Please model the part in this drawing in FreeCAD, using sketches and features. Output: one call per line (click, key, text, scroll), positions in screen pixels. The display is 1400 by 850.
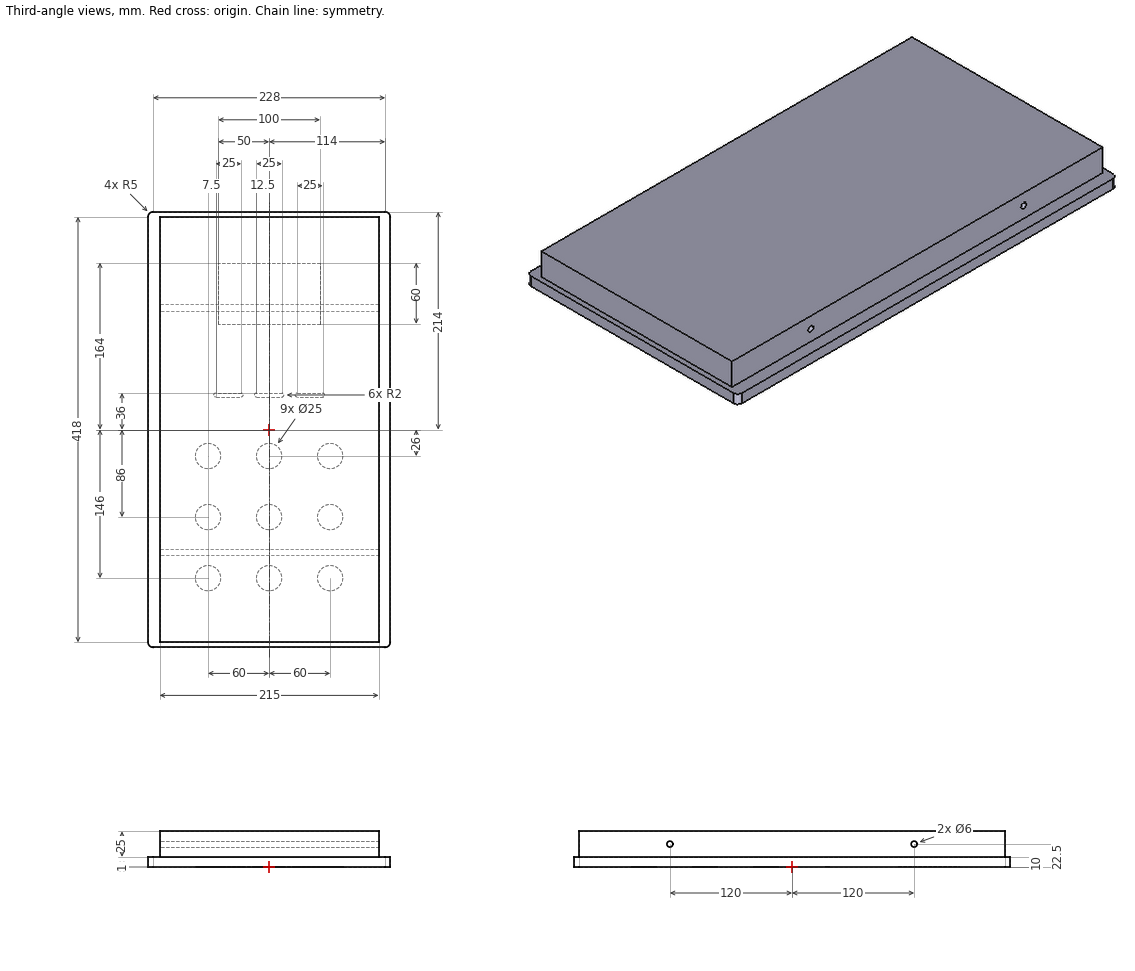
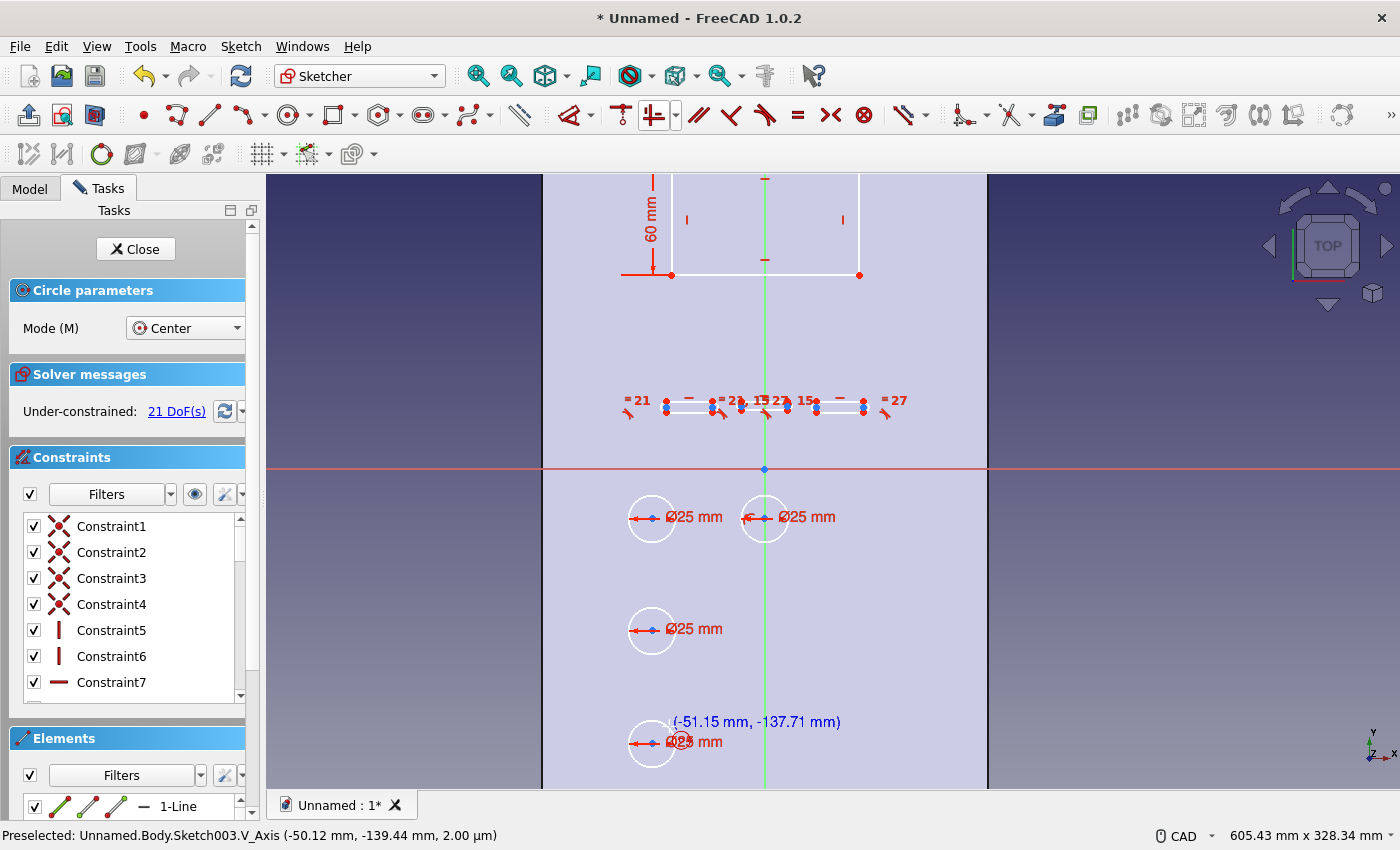
click(765, 630)
move(781, 614)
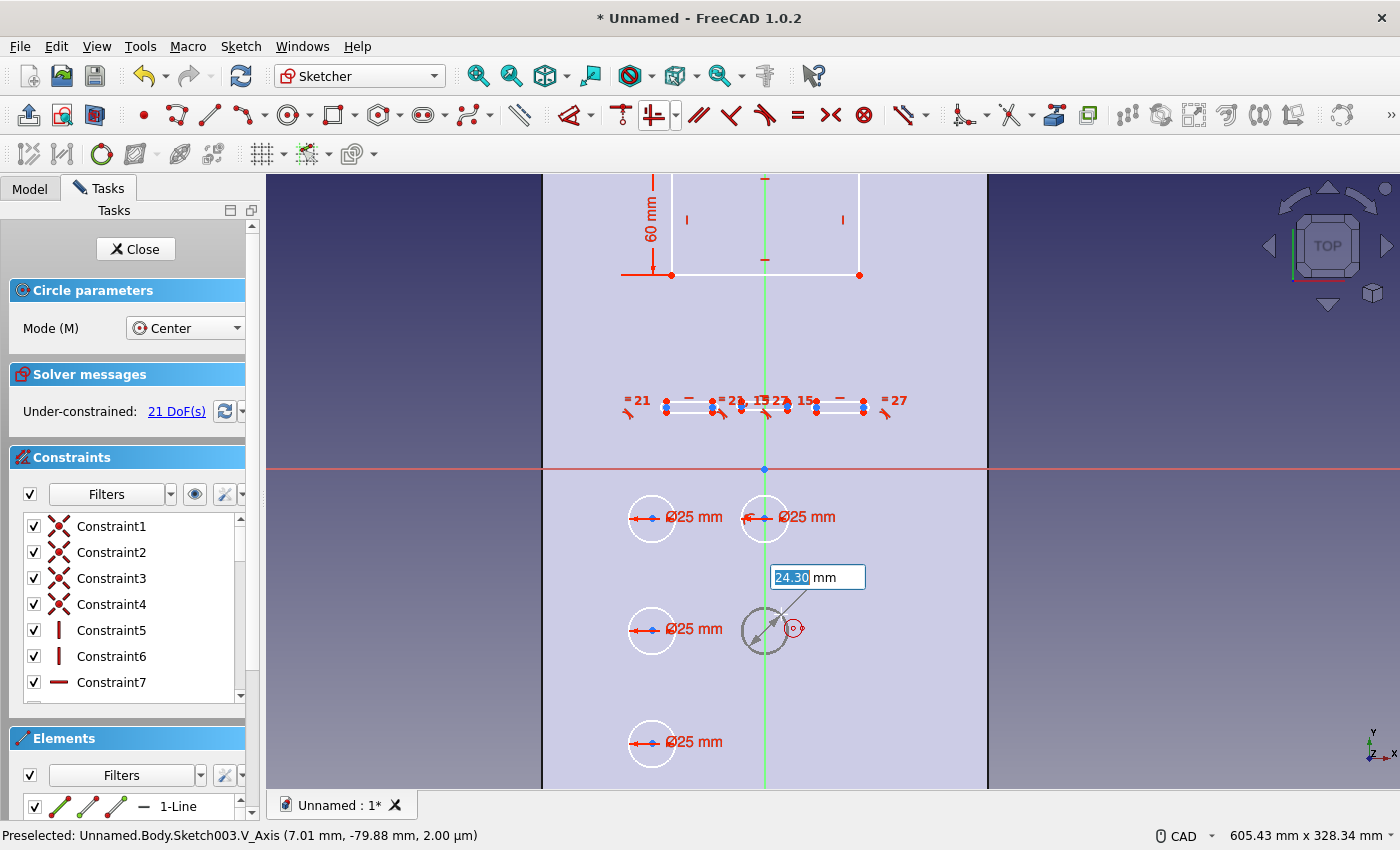
text(25)
key(Return)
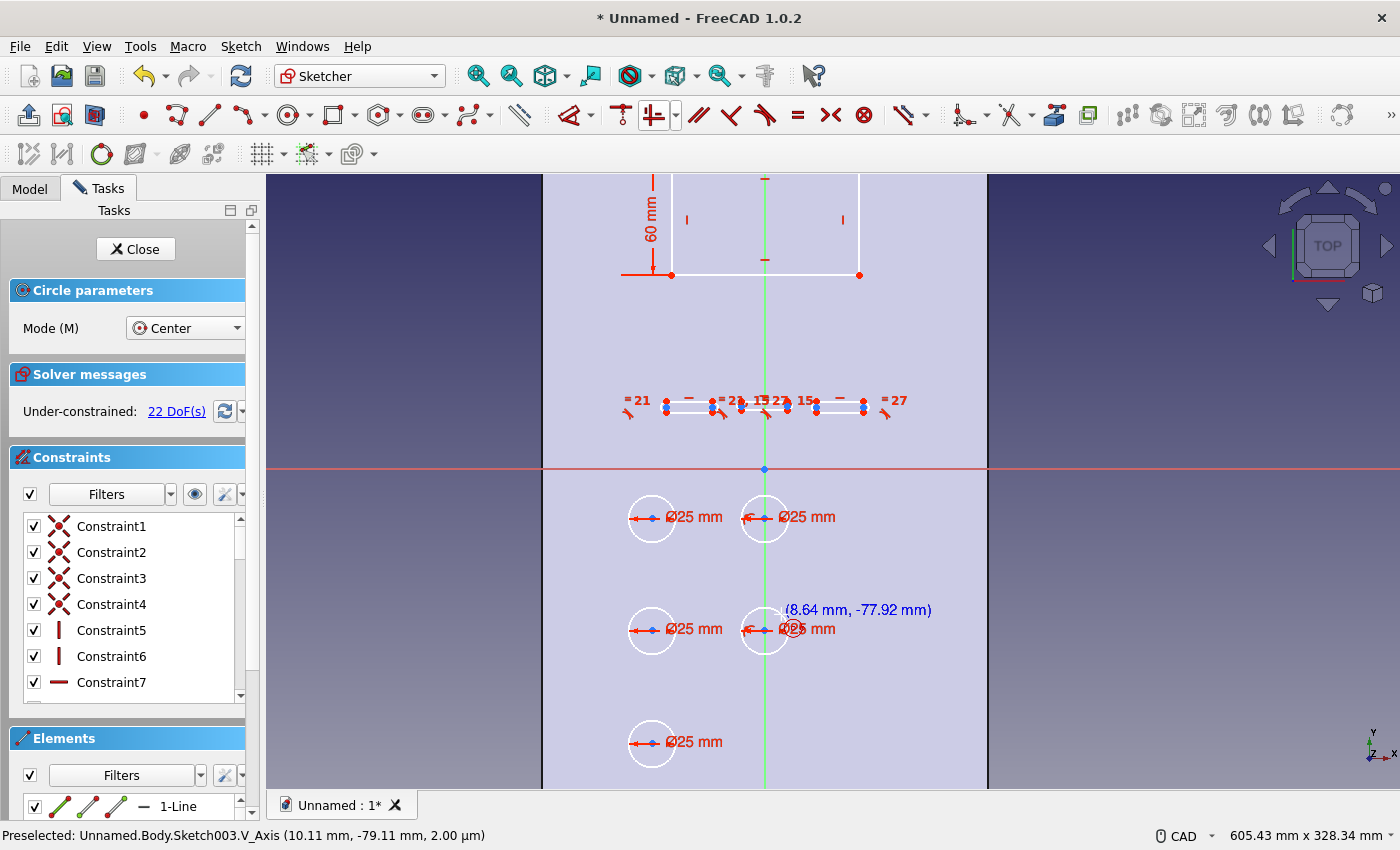
click(765, 743)
move(781, 726)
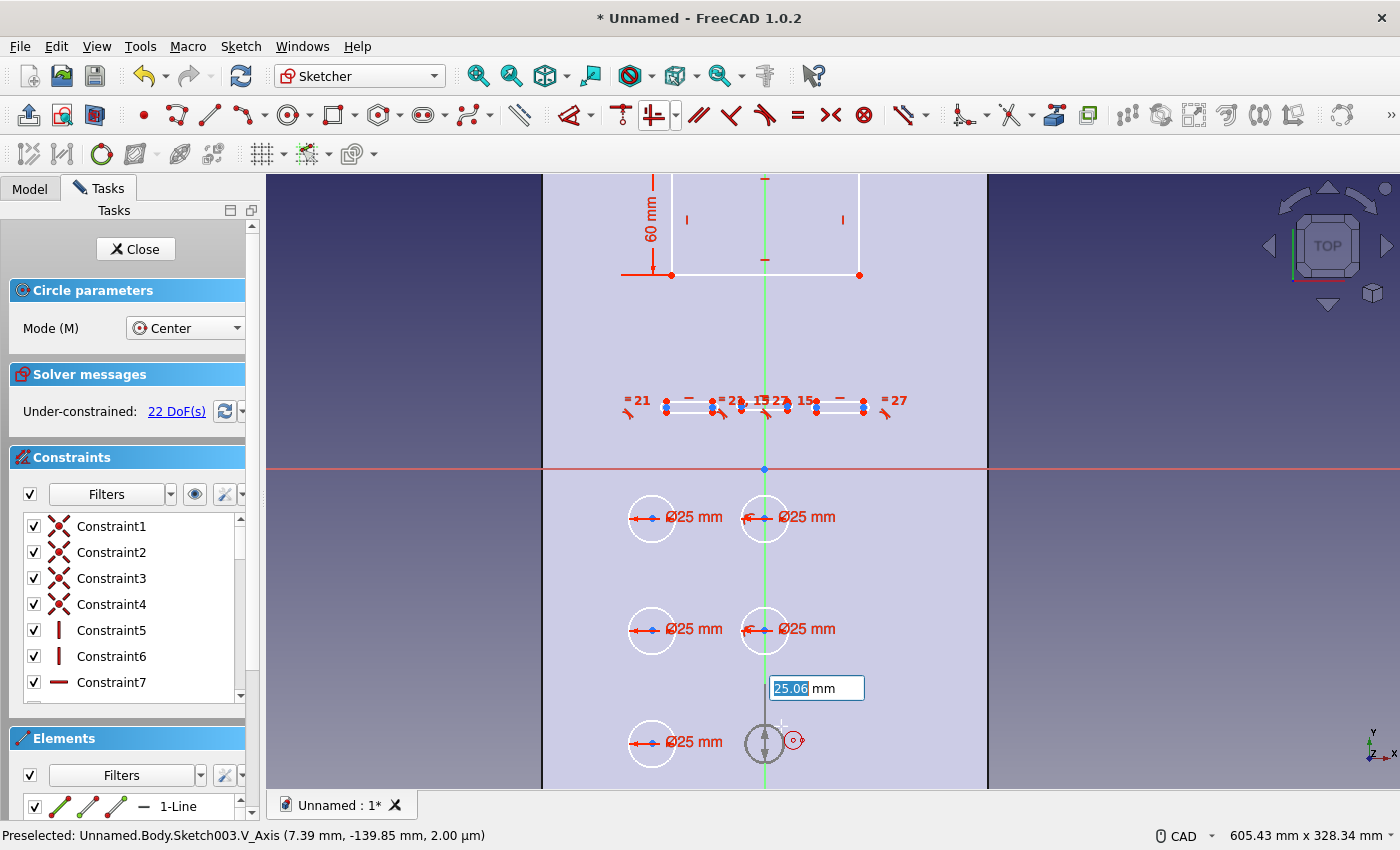
text(25)
key(Return)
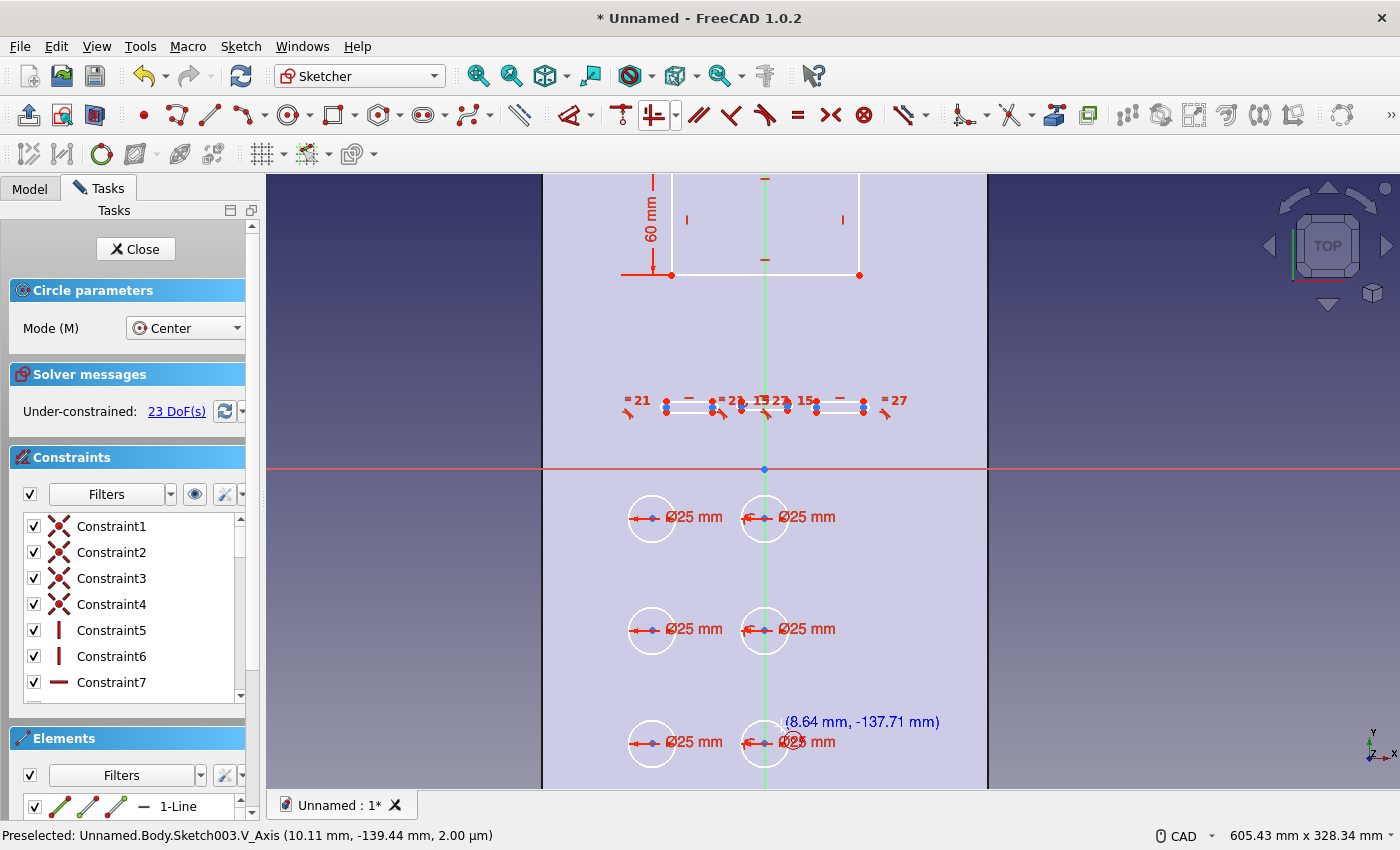
click(877, 743)
move(894, 726)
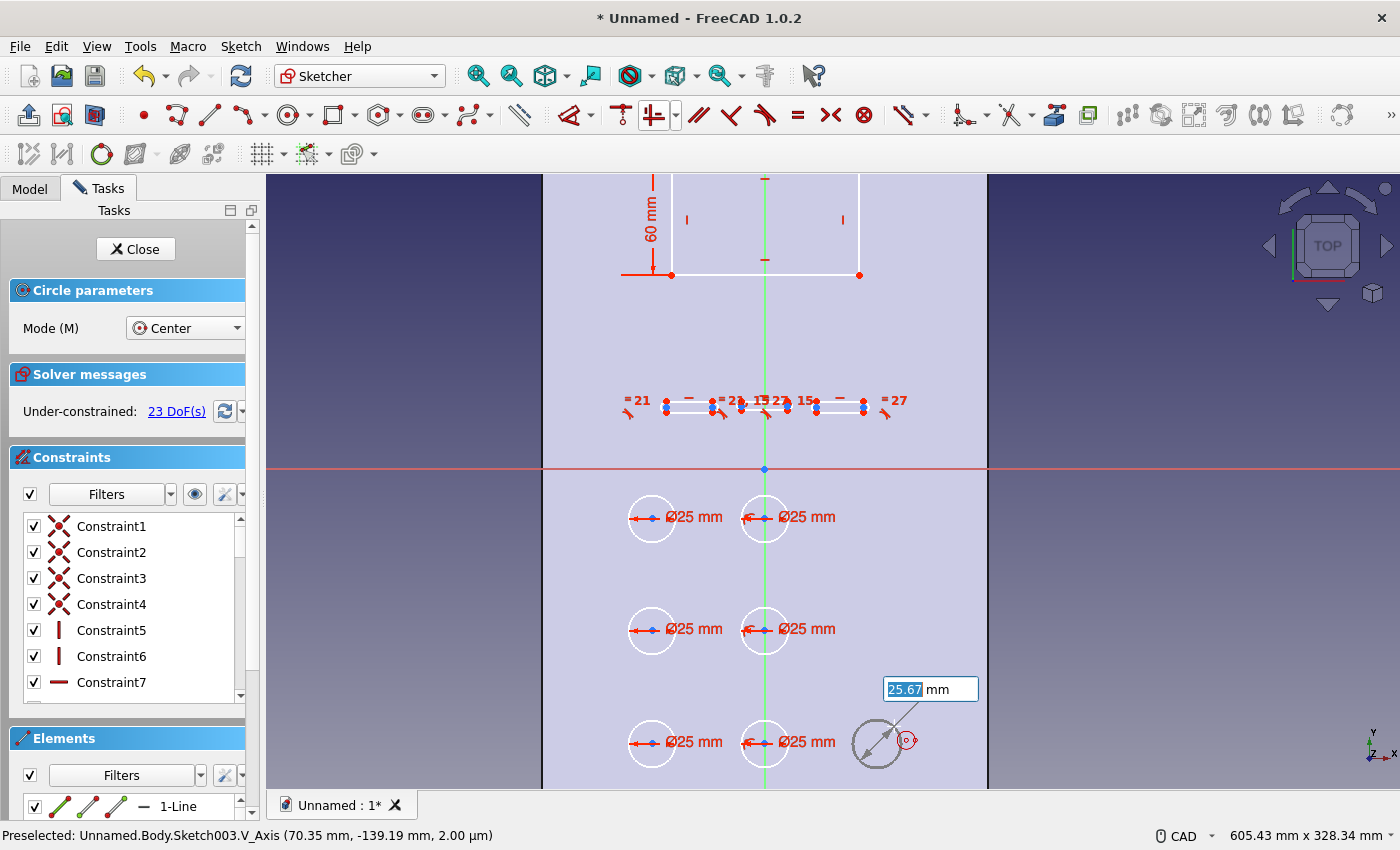
text(25)
key(Return)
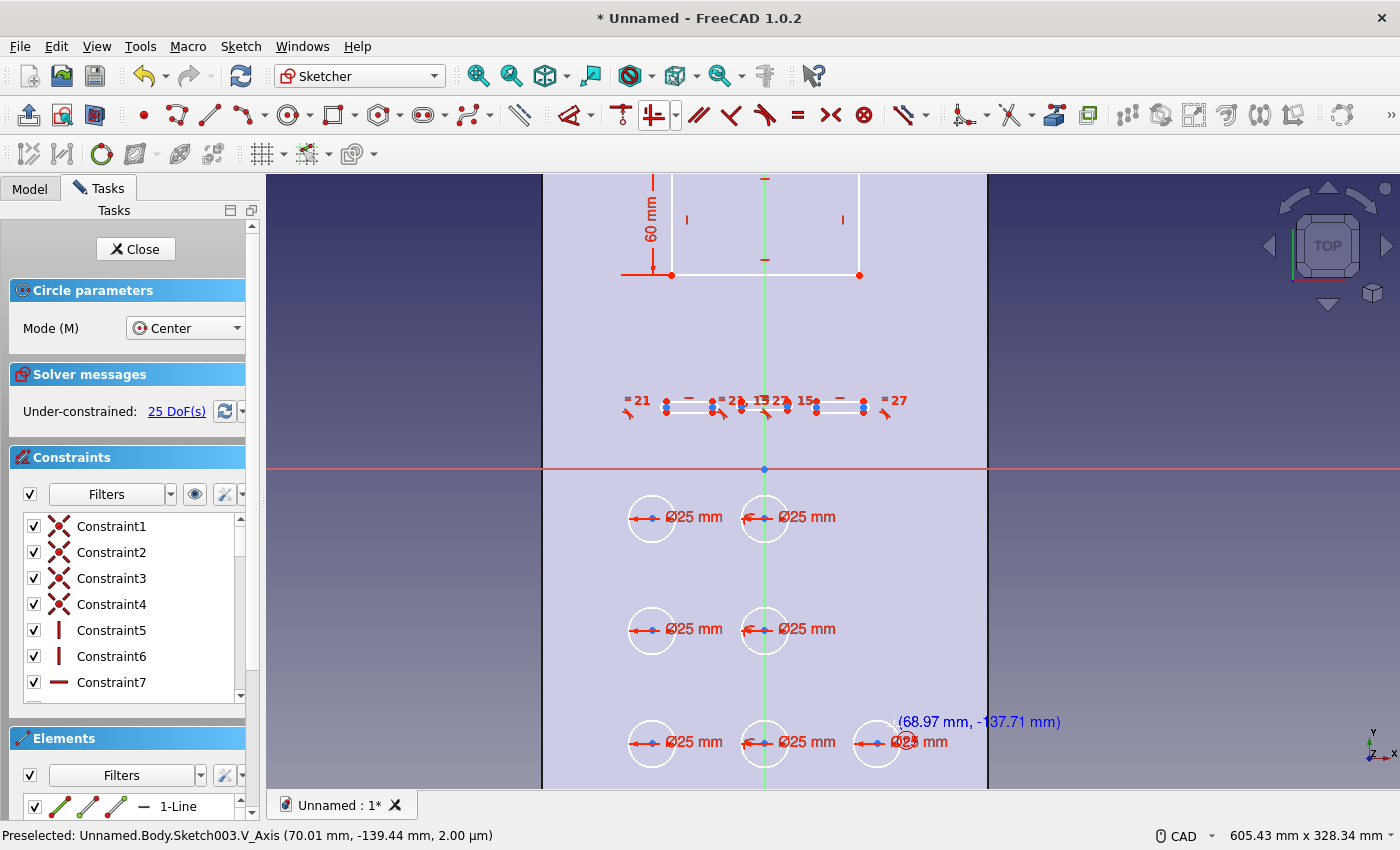
click(877, 630)
move(894, 614)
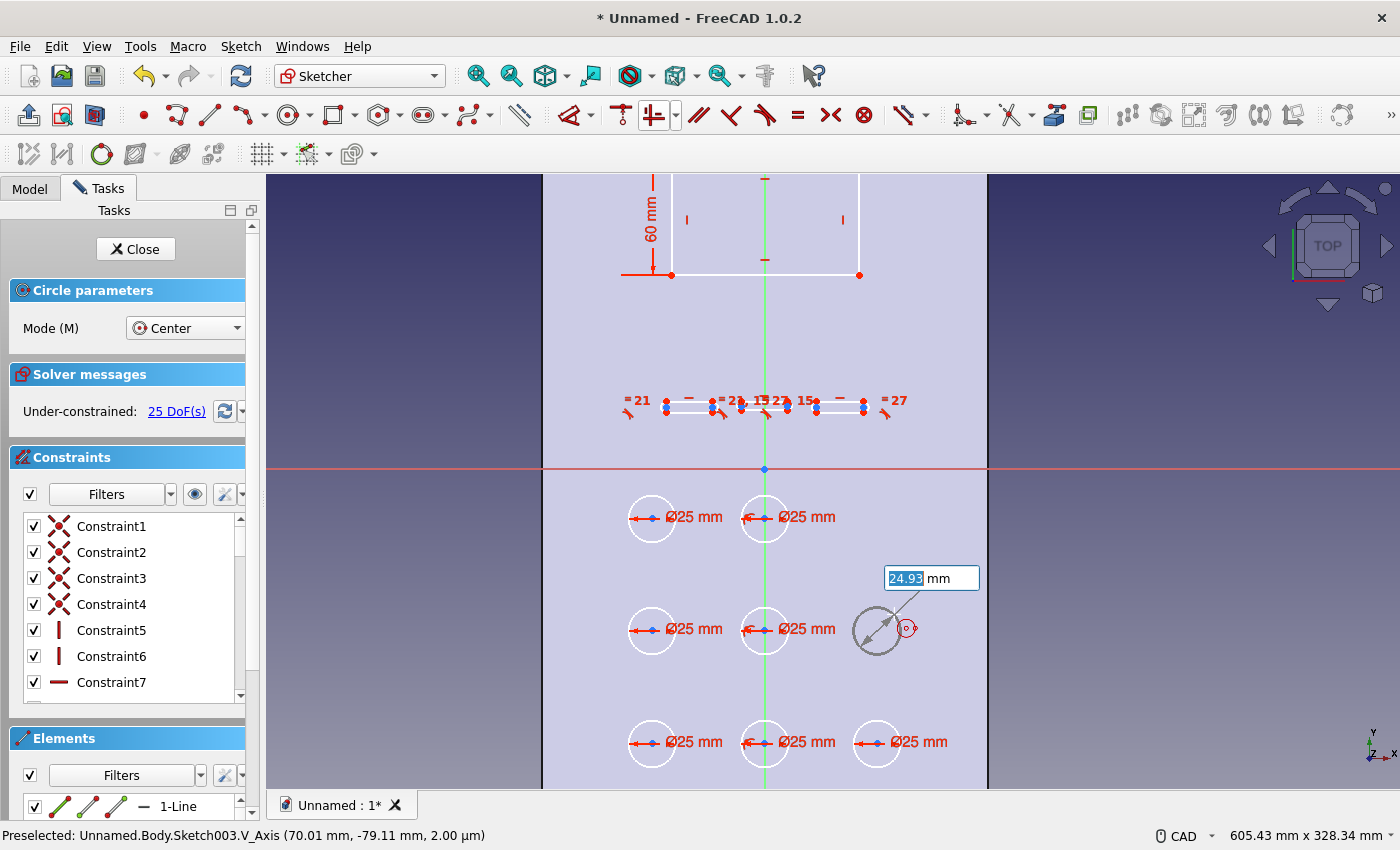
text(25)
key(Return)